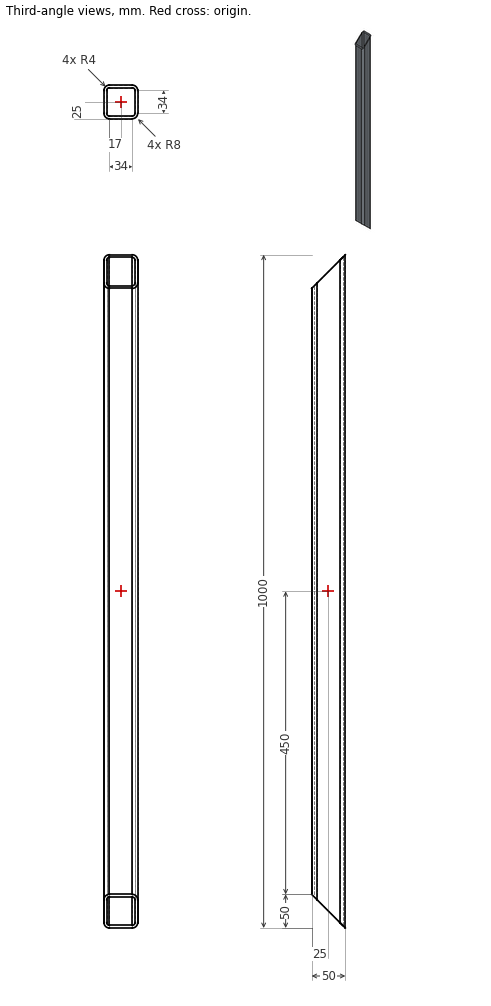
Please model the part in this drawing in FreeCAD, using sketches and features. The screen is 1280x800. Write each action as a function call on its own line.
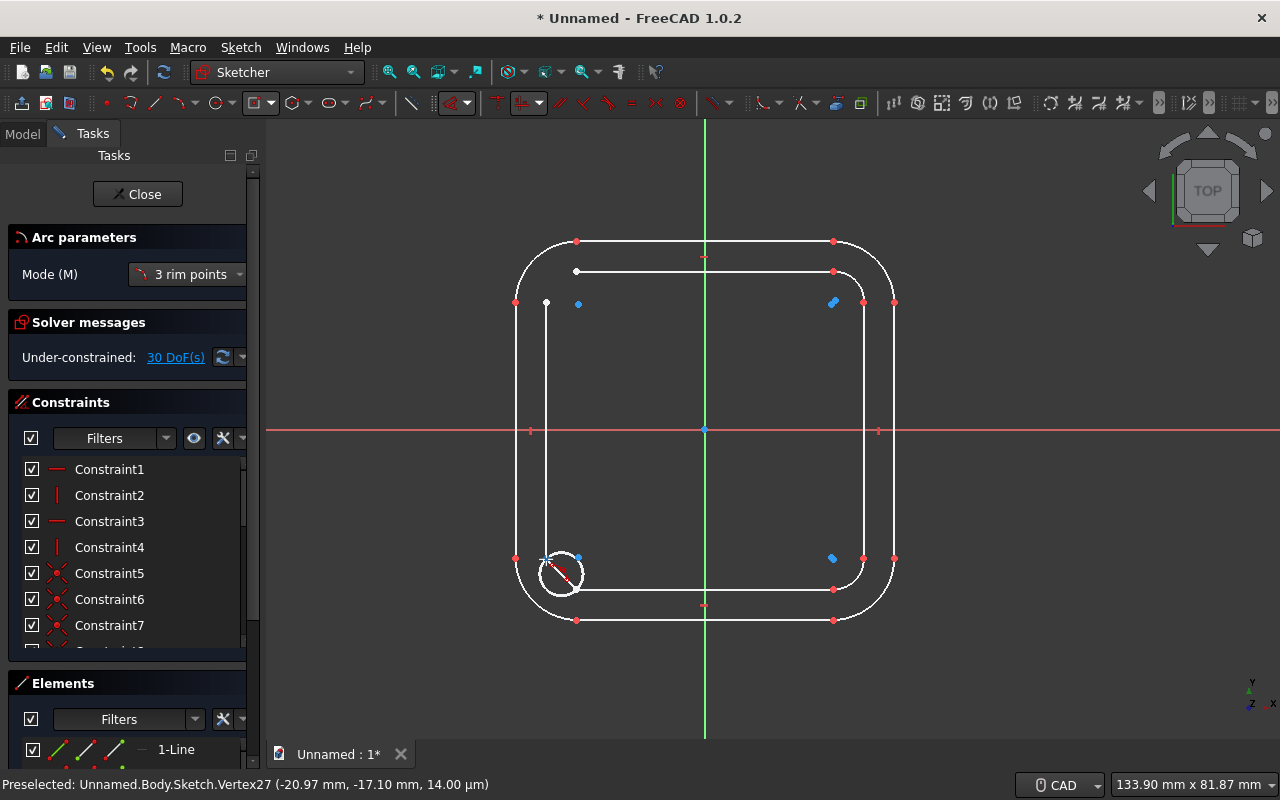
scroll(555, 580, up, 3)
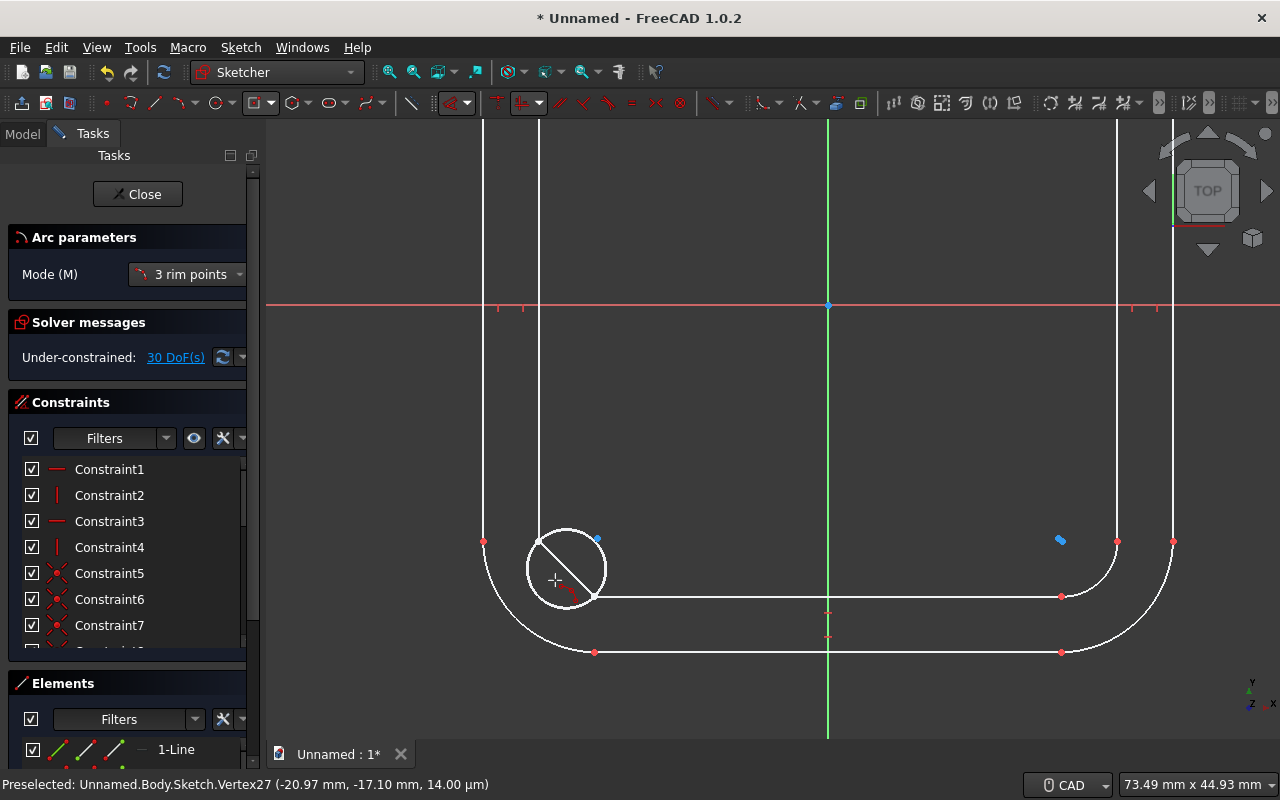
click(554, 579)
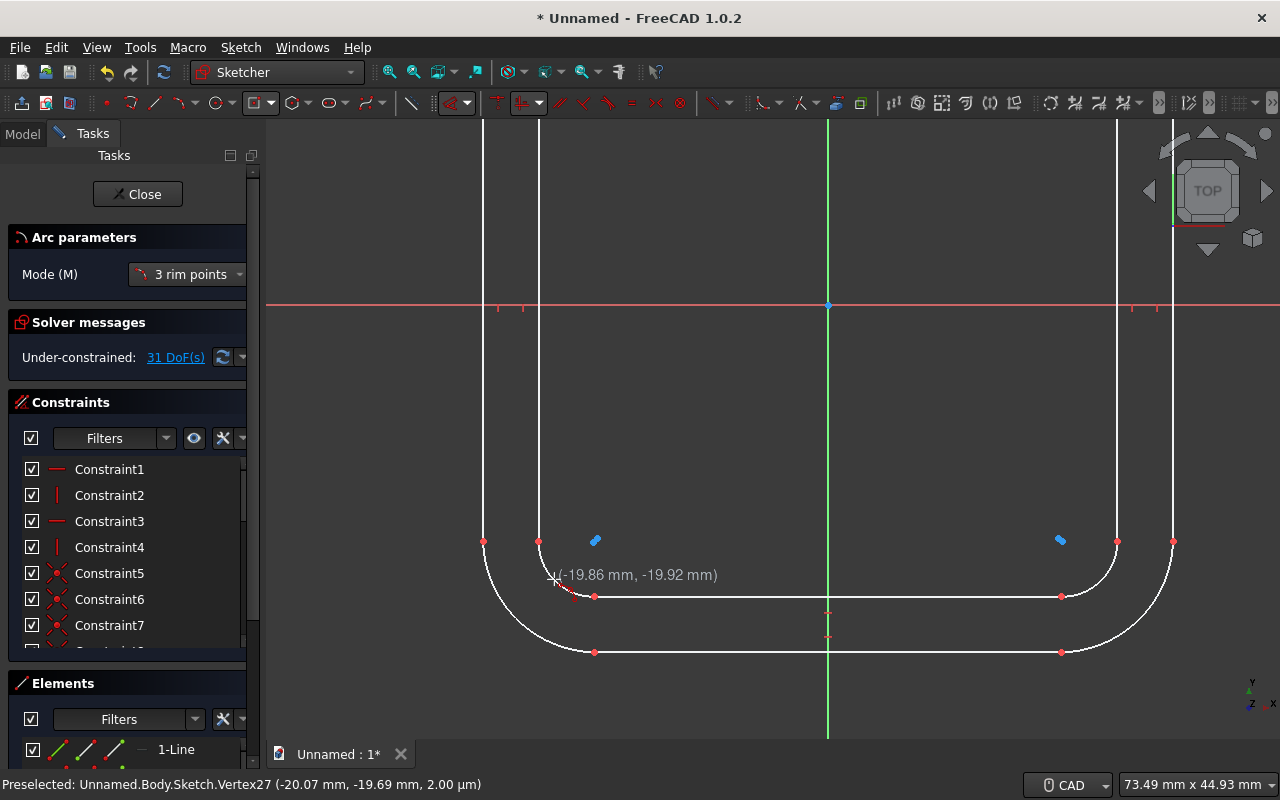
scroll(554, 580, down, 3)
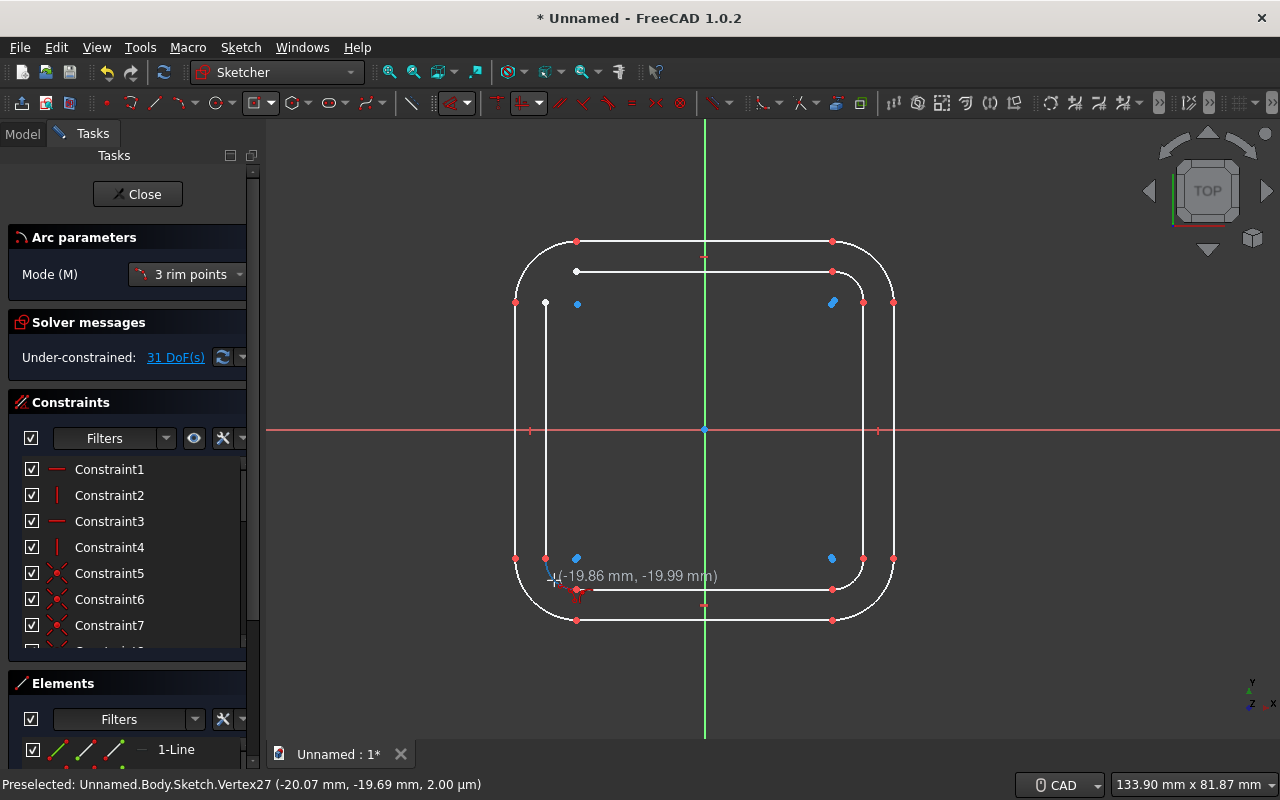
click(546, 302)
click(576, 272)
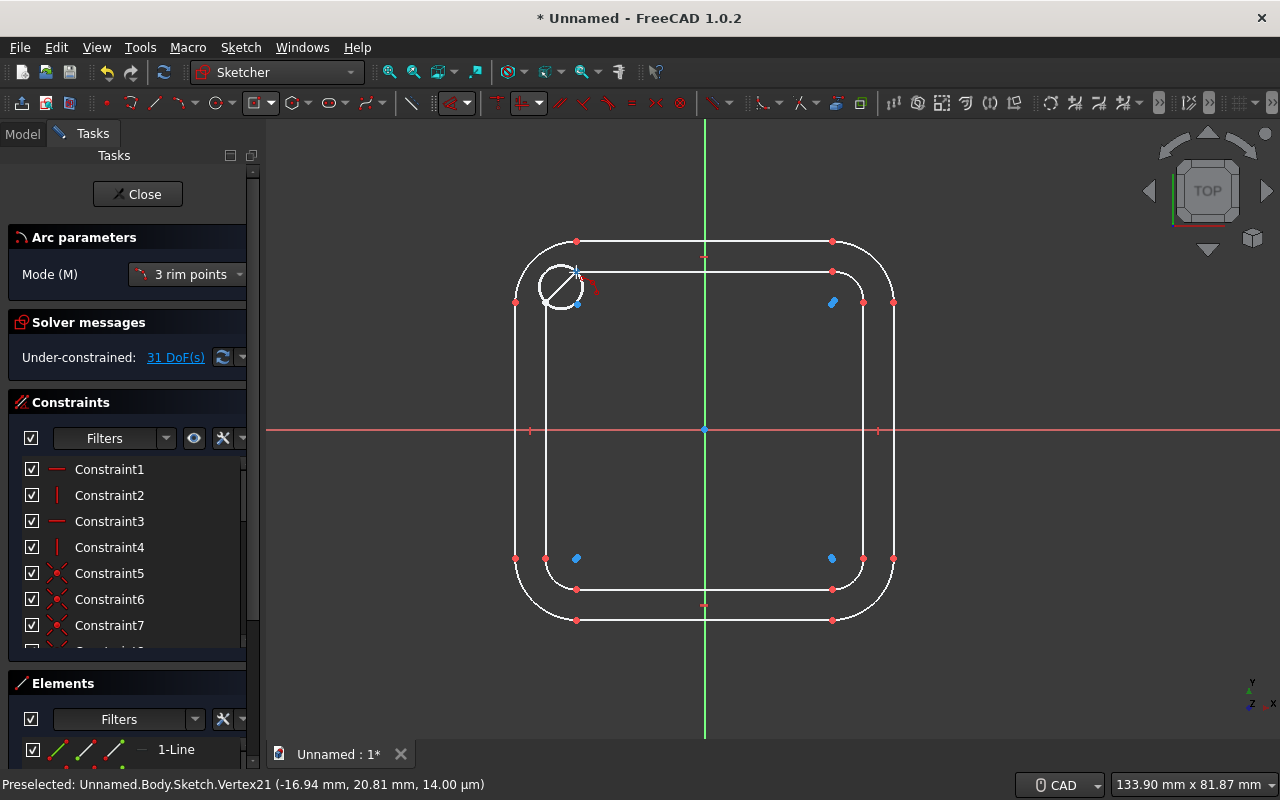
scroll(554, 279, up, 3)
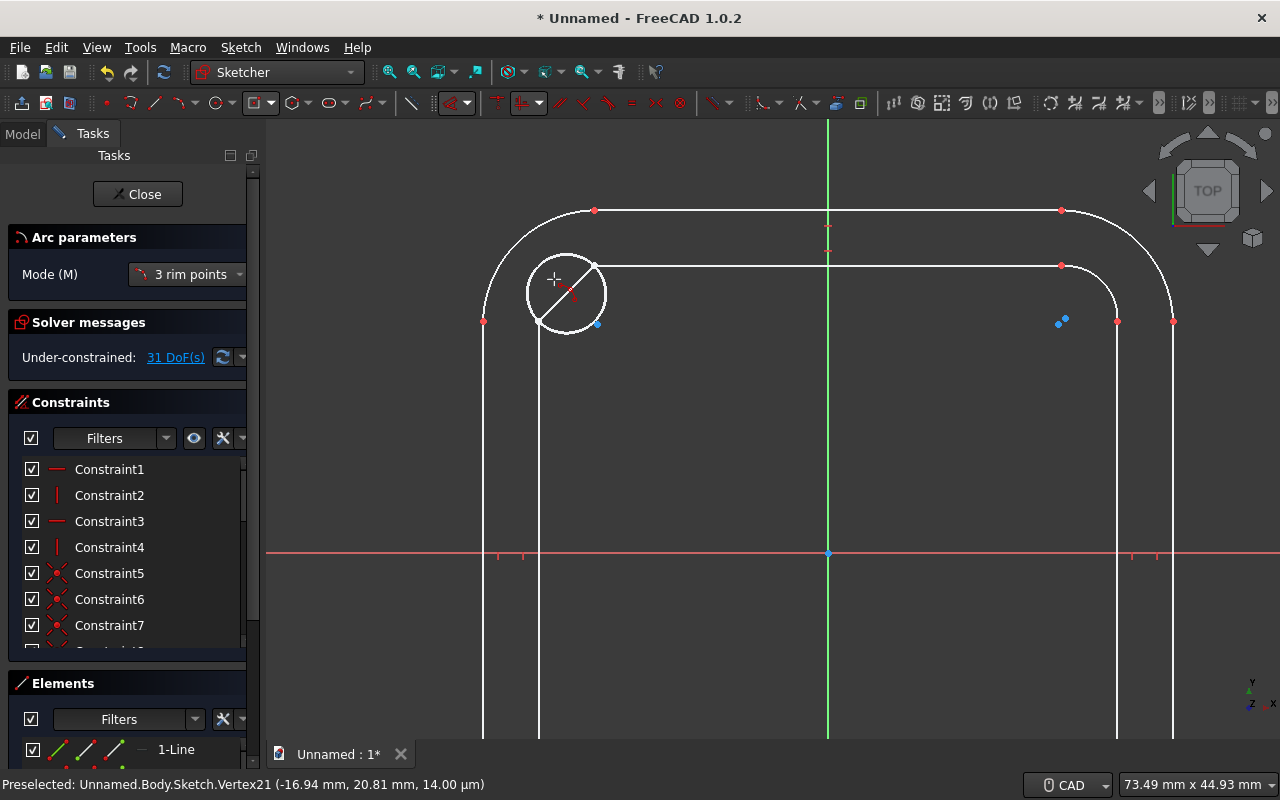
click(554, 279)
key(Escape)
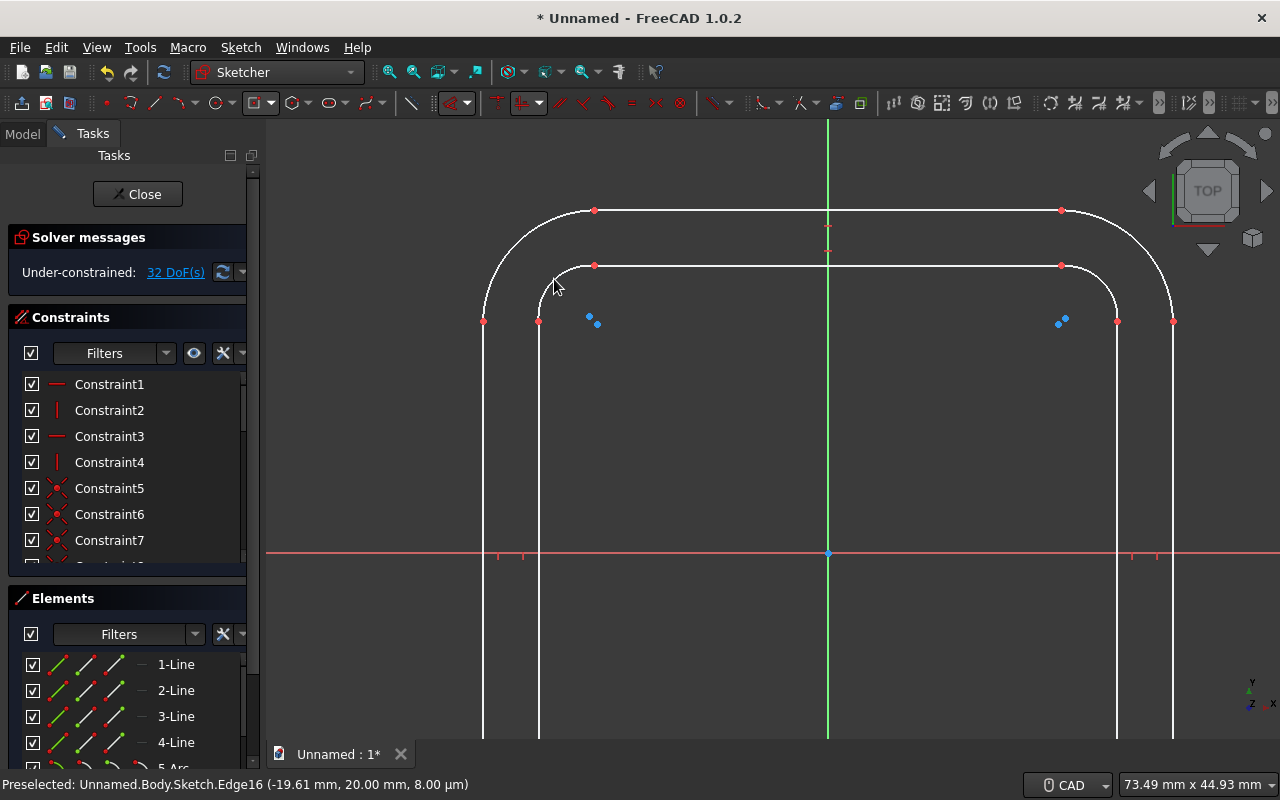
scroll(554, 278, down, 3)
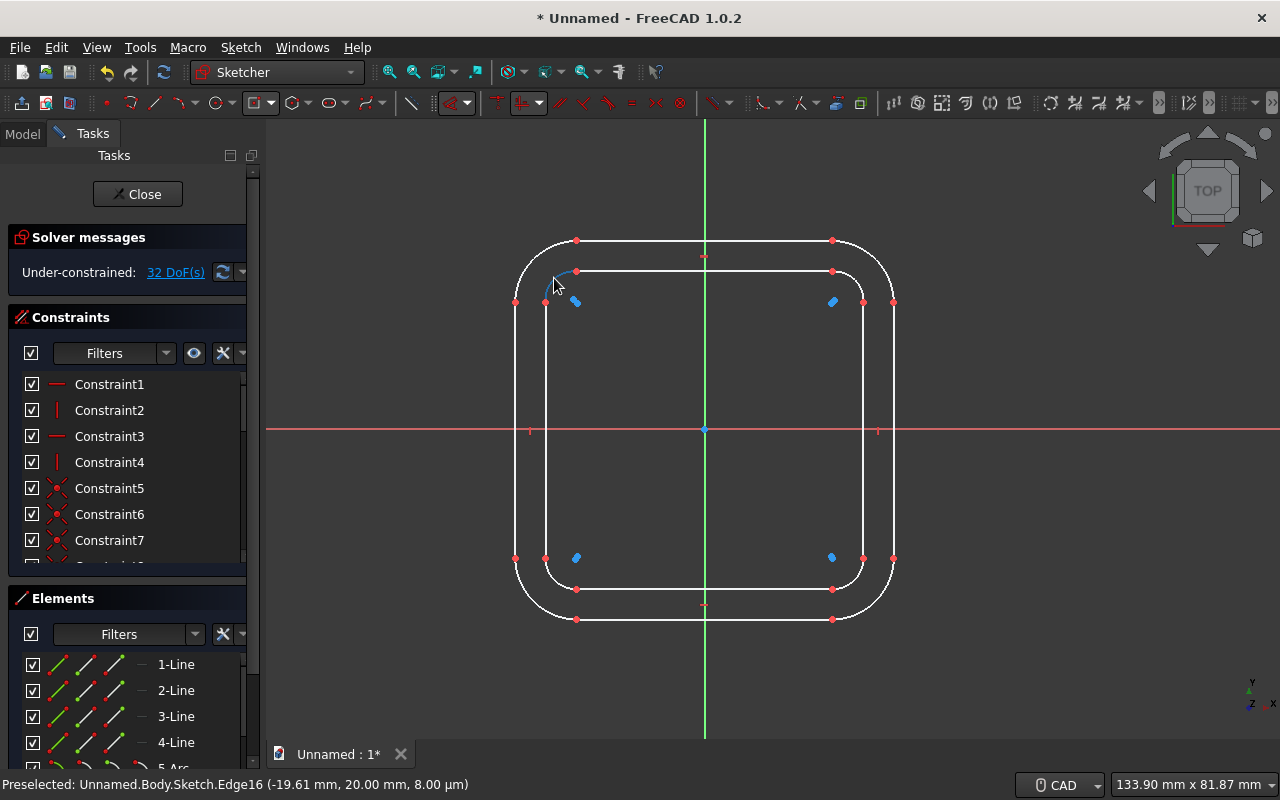
click(653, 620)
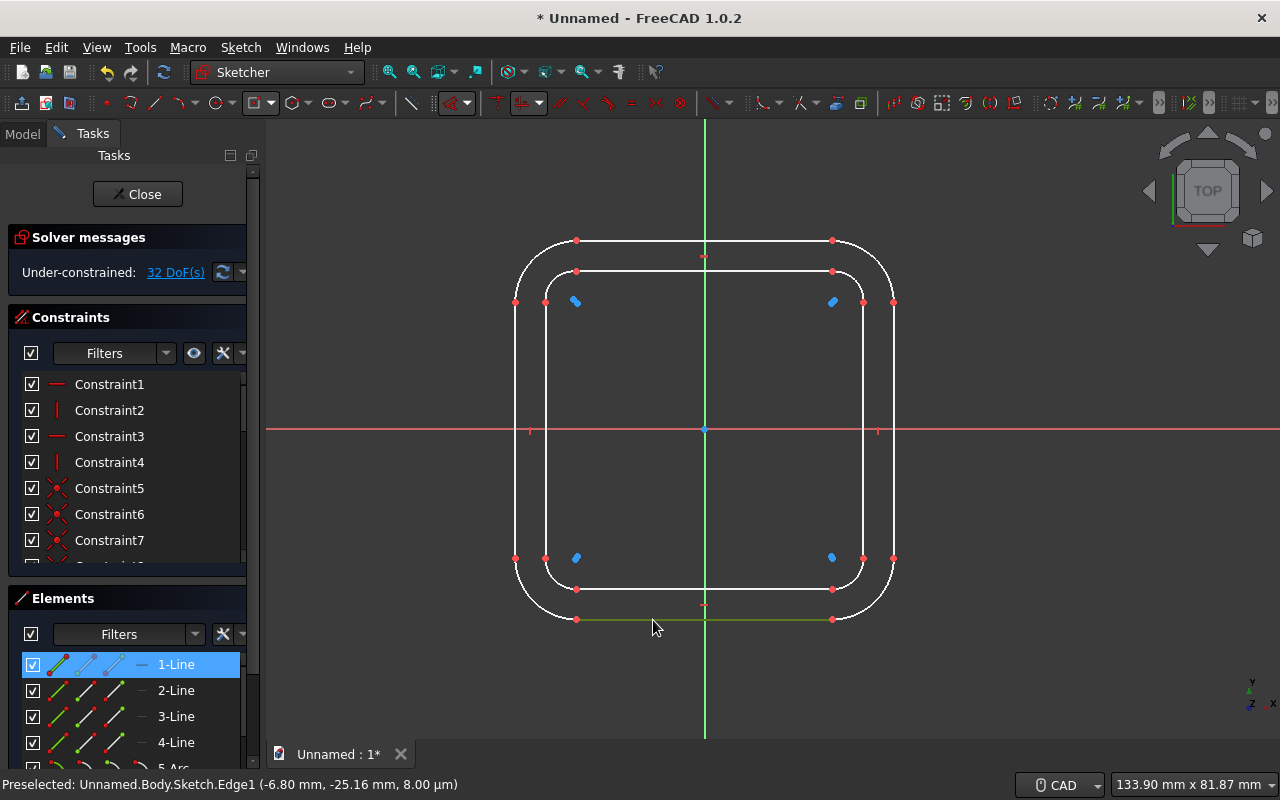
click(860, 613)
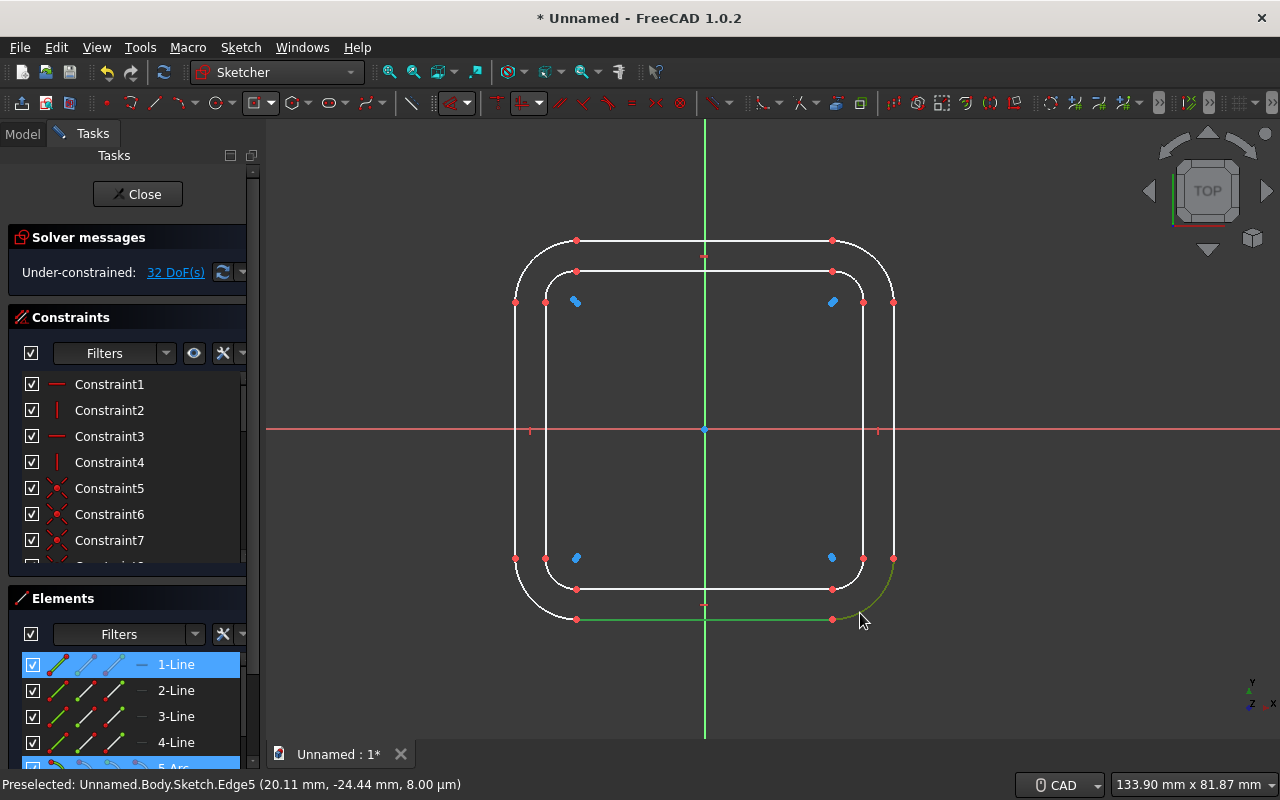
key(t)